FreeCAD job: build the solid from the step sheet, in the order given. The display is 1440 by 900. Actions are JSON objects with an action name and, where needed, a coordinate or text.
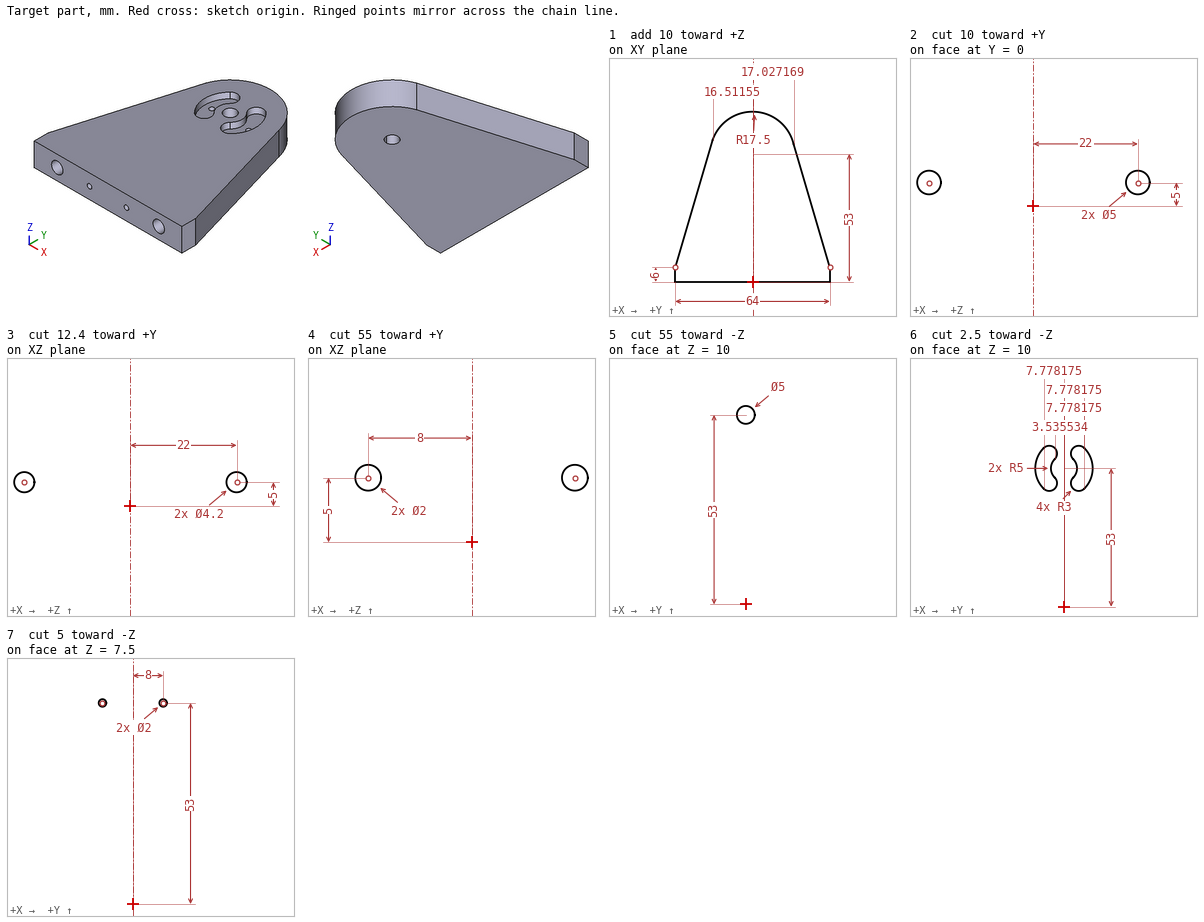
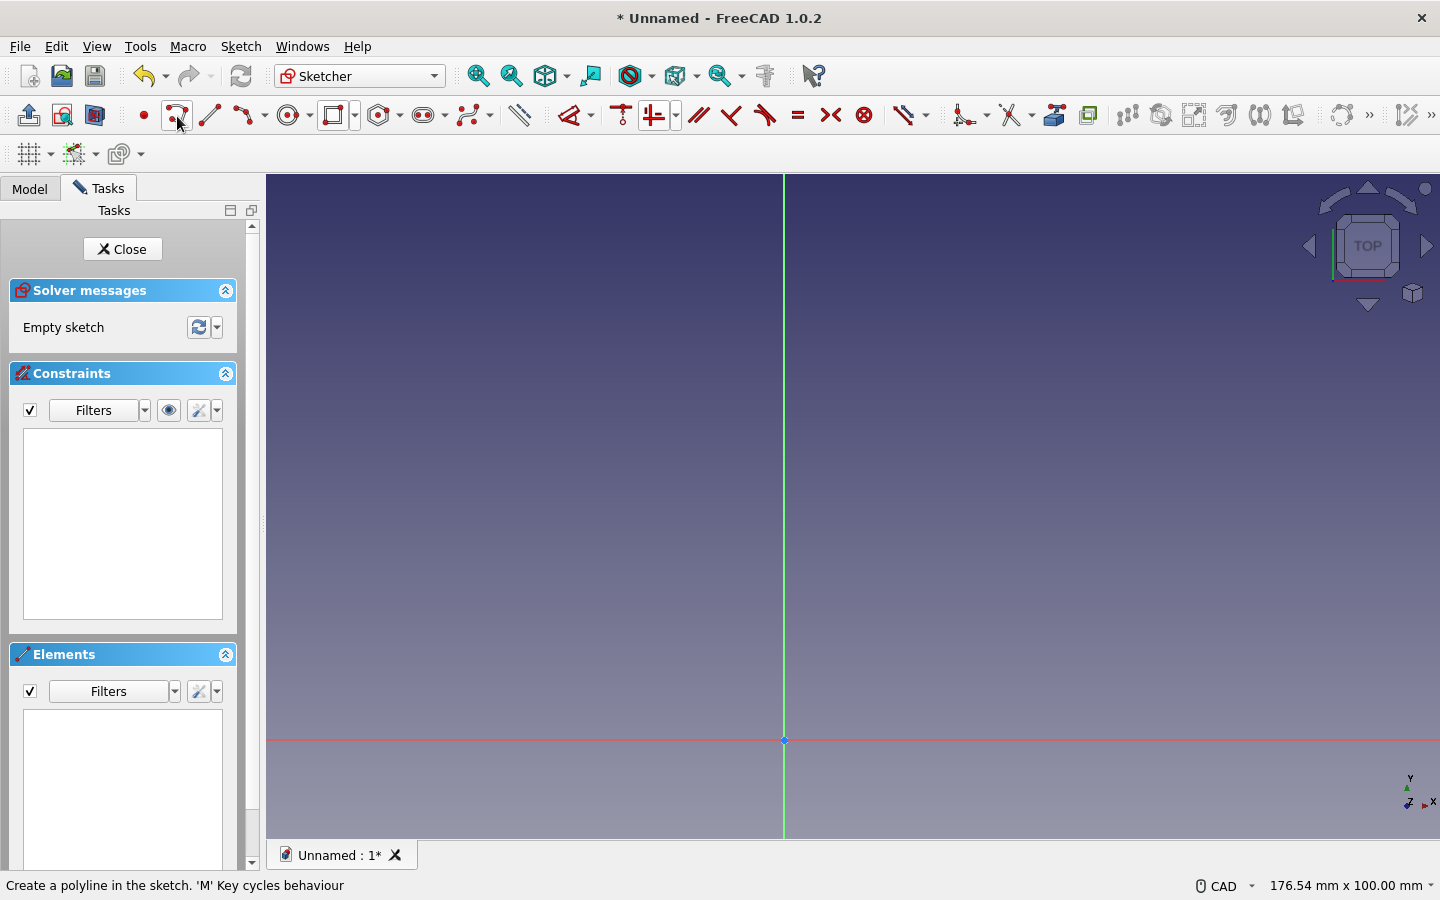
{"action": "left_click", "coordinate": [674, 349]}
{"action": "left_click", "coordinate": [571, 701]}
{"action": "left_click", "coordinate": [571, 740]}
{"action": "left_click", "coordinate": [997, 731]}
{"action": "left_click", "coordinate": [997, 701]}
{"action": "left_click", "coordinate": [897, 361]}
{"action": "right_click", "coordinate": [897, 361]}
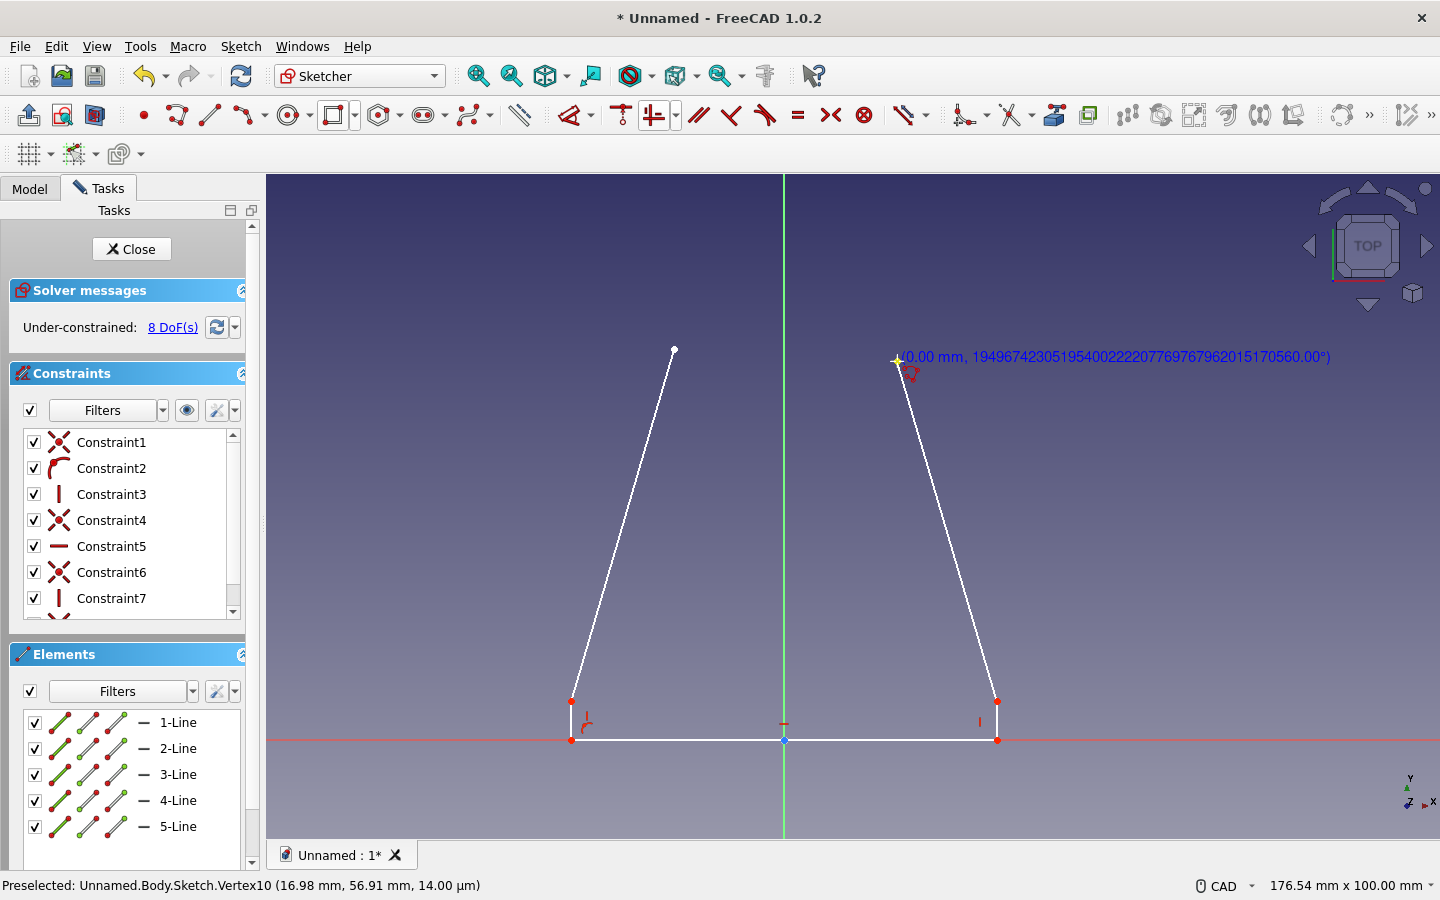
{"action": "left_click", "coordinate": [242, 116]}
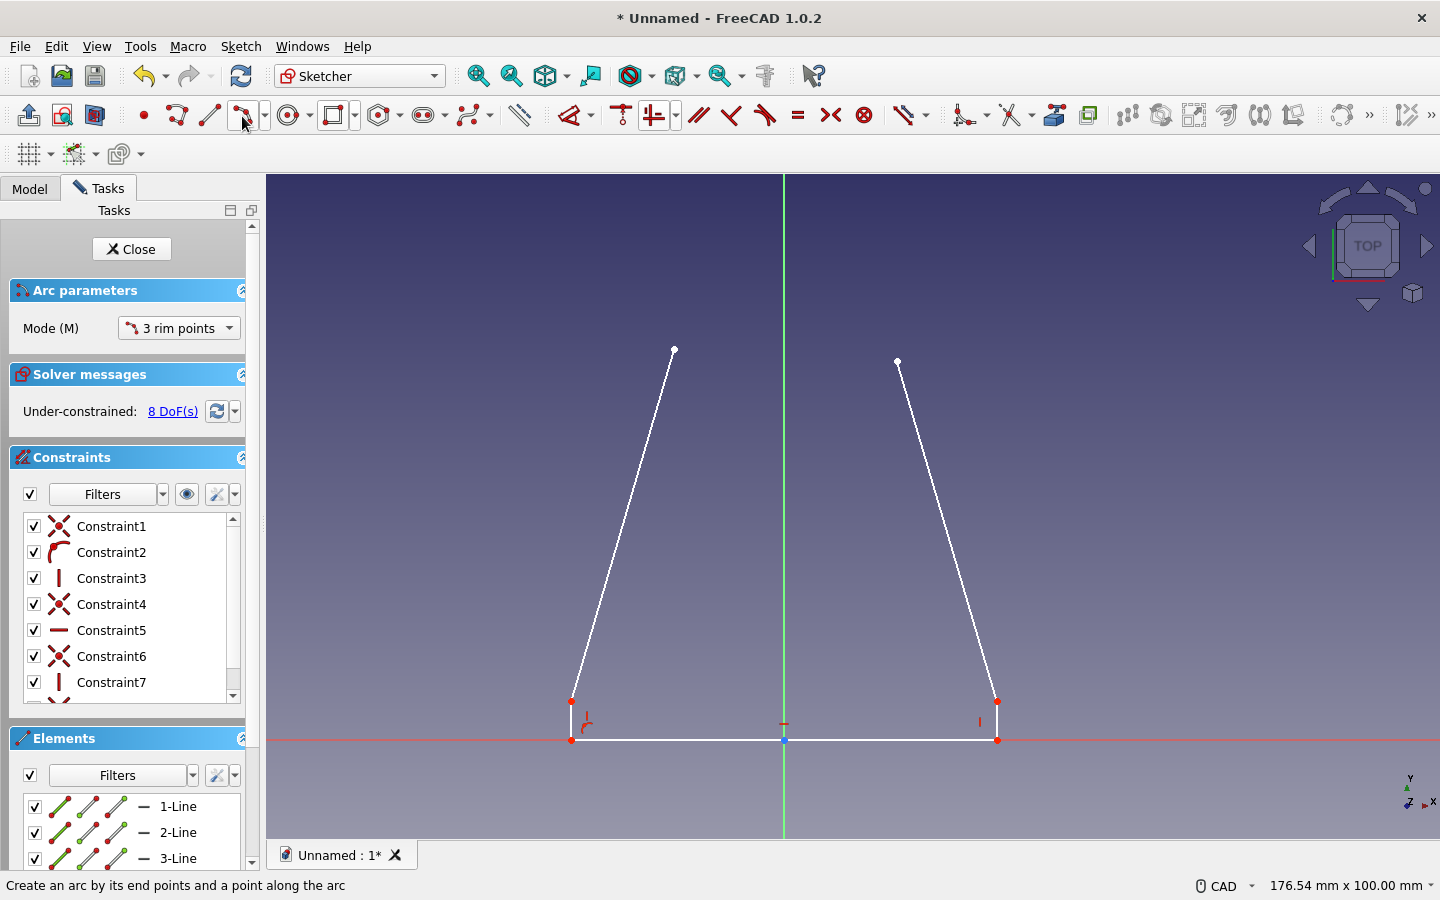
{"action": "left_click", "coordinate": [897, 362]}
{"action": "left_click", "coordinate": [674, 350]}
{"action": "left_click", "coordinate": [820, 277]}
{"action": "key", "text": "Escape"}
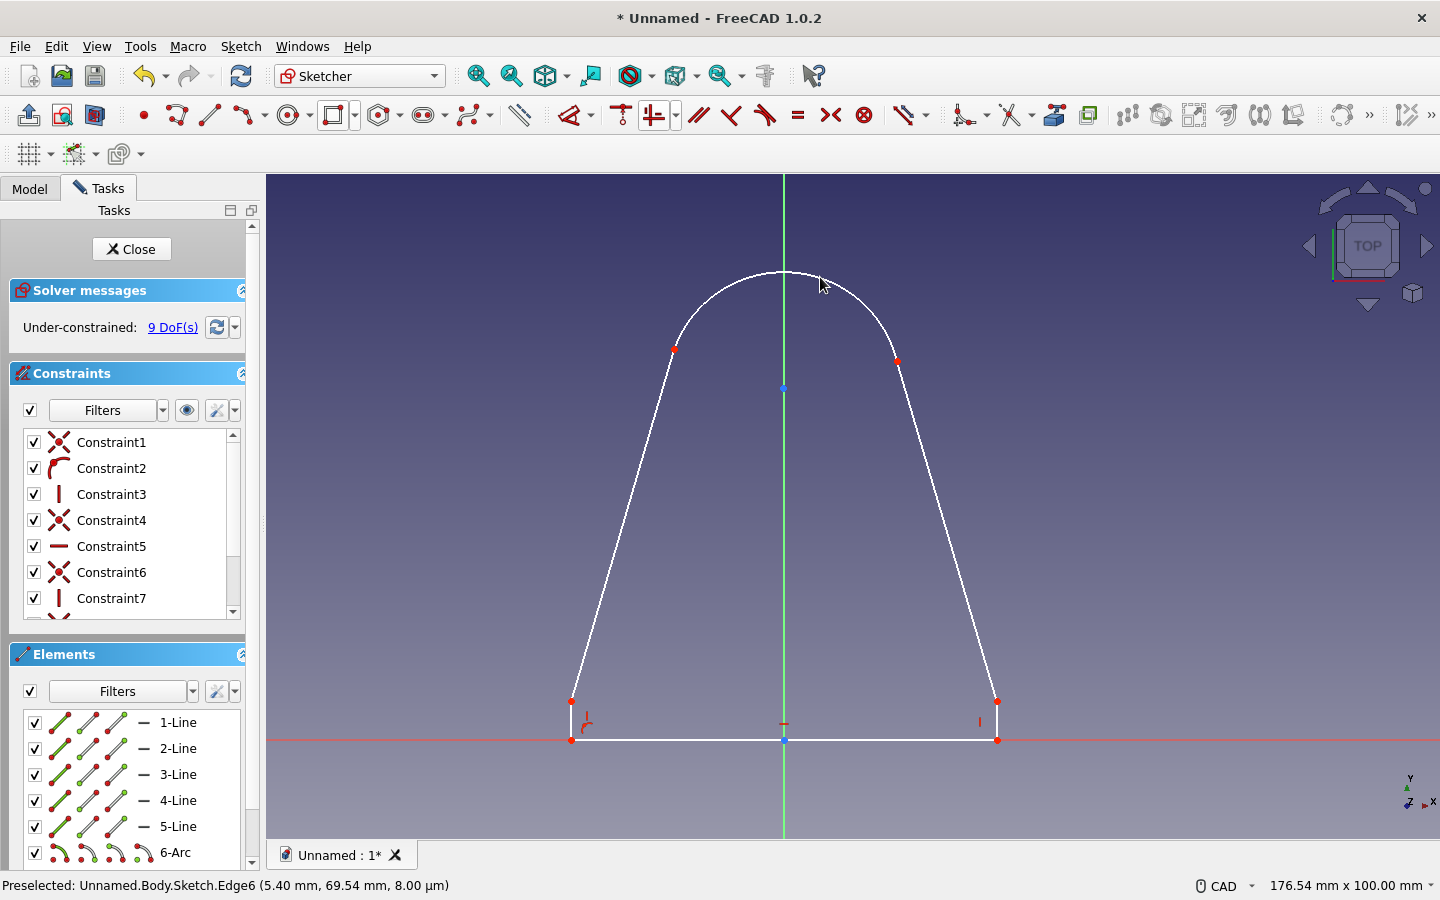
{"action": "left_click", "coordinate": [784, 389]}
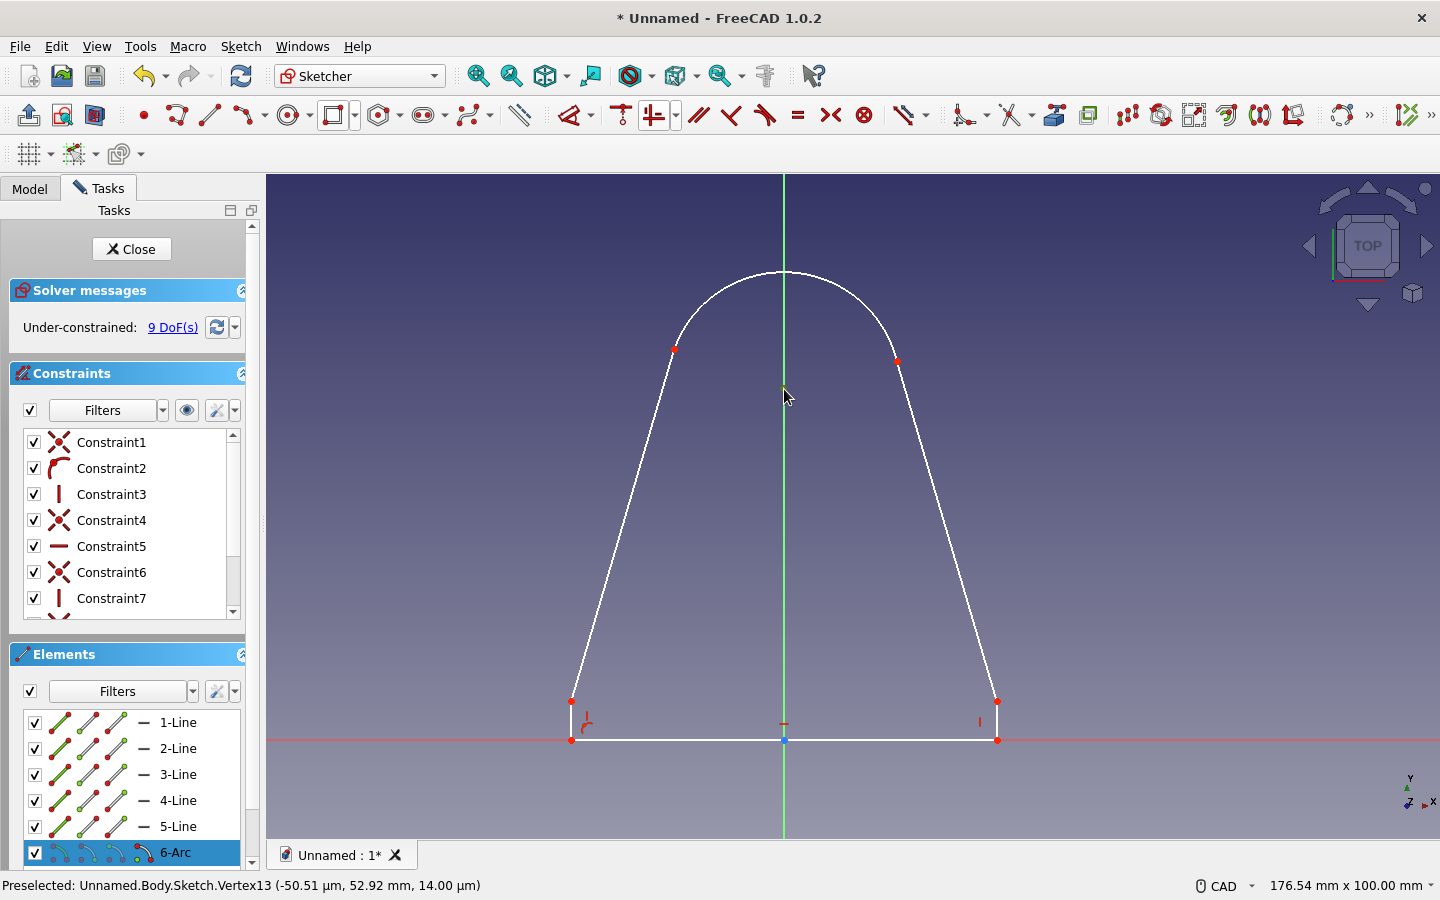
{"action": "left_click", "coordinate": [784, 680]}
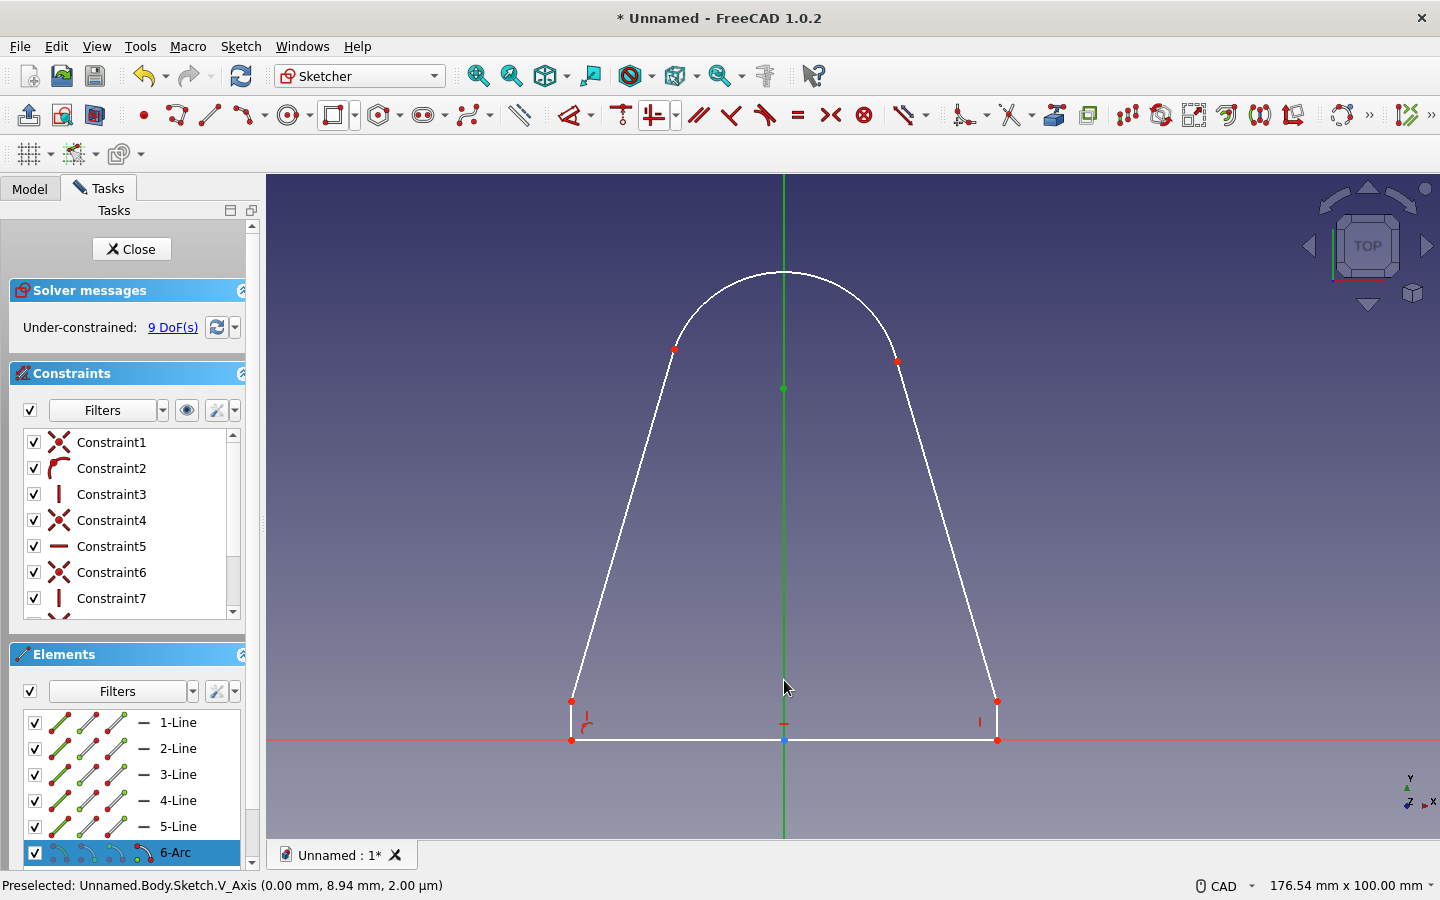
{"action": "left_click", "coordinate": [621, 116]}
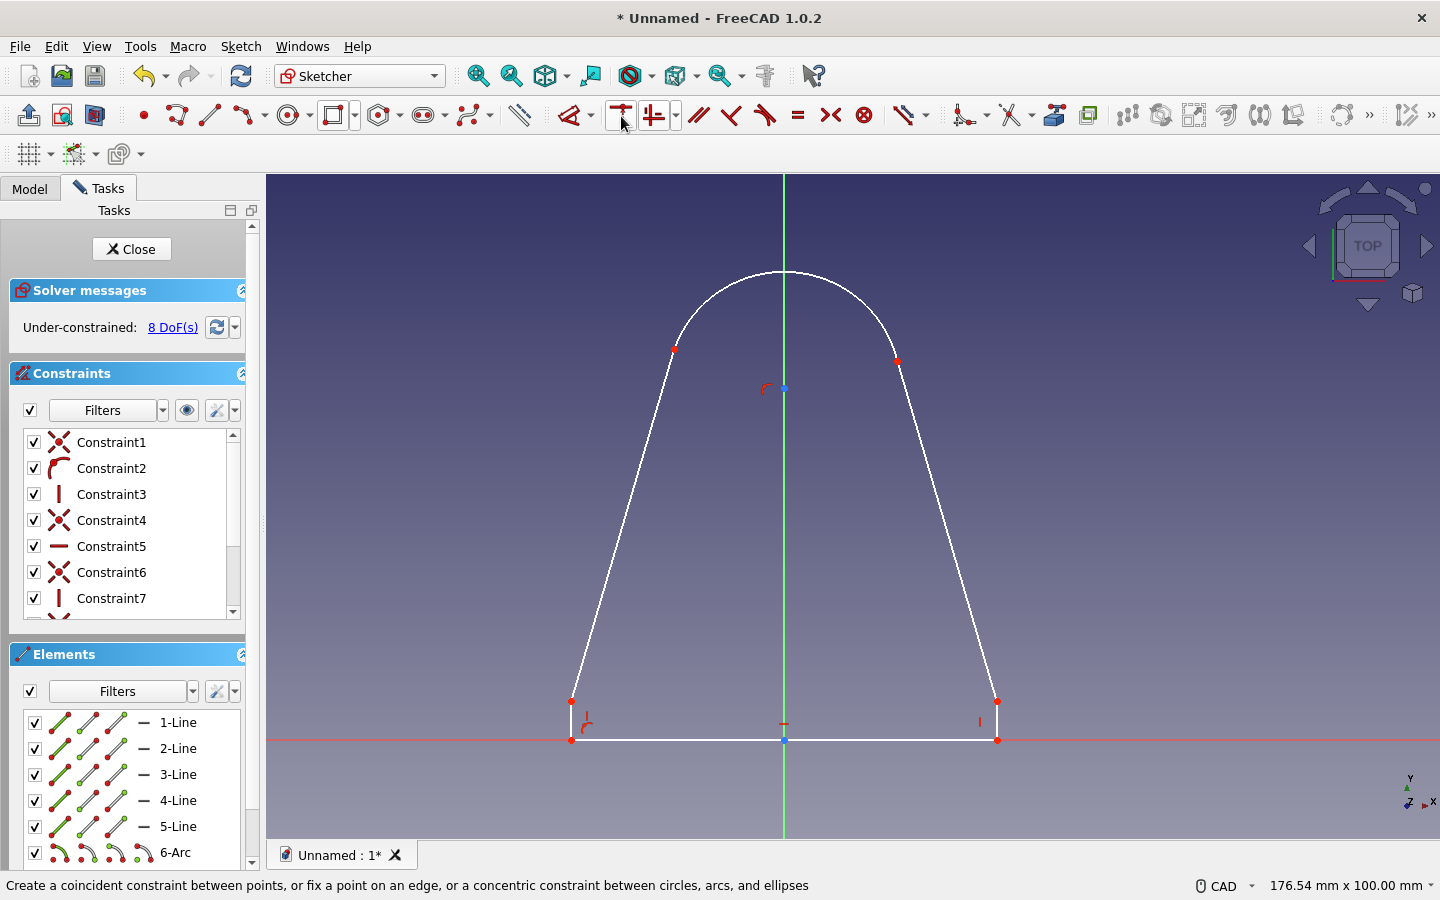
{"action": "left_click", "coordinate": [571, 702]}